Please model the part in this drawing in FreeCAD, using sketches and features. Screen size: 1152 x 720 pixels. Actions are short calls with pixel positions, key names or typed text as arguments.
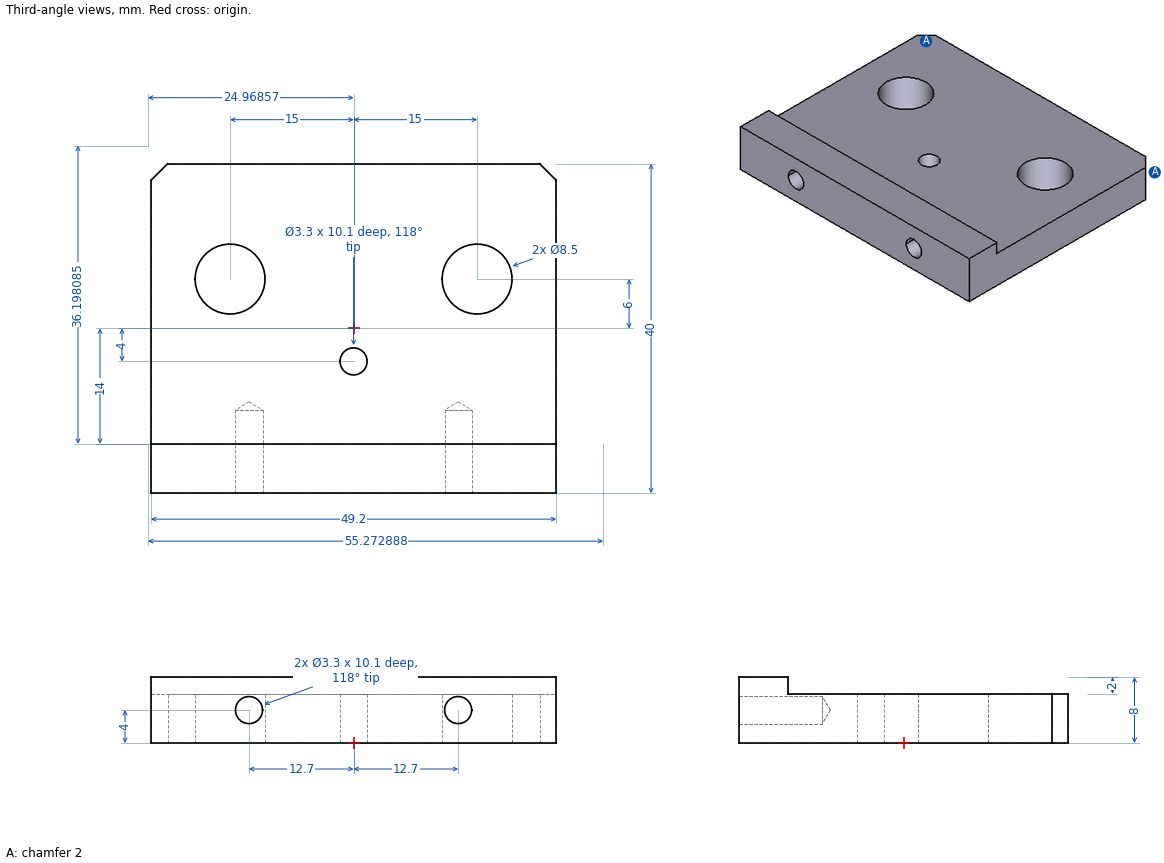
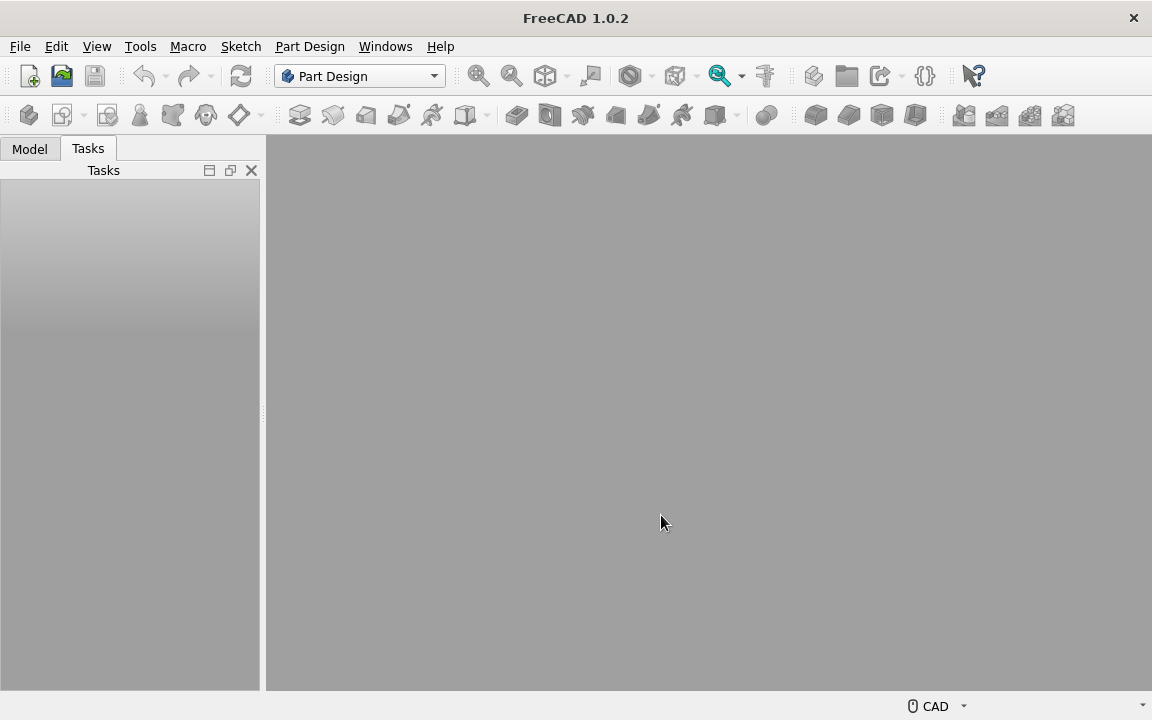
key(ctrl+n)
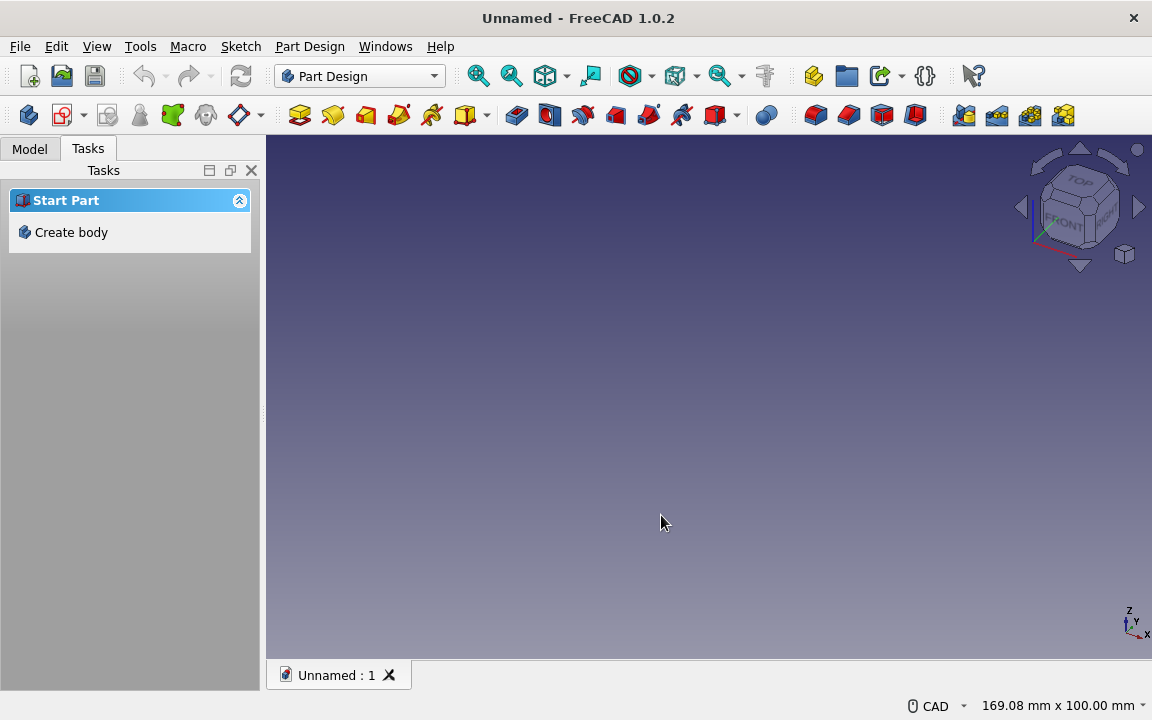
click(62, 116)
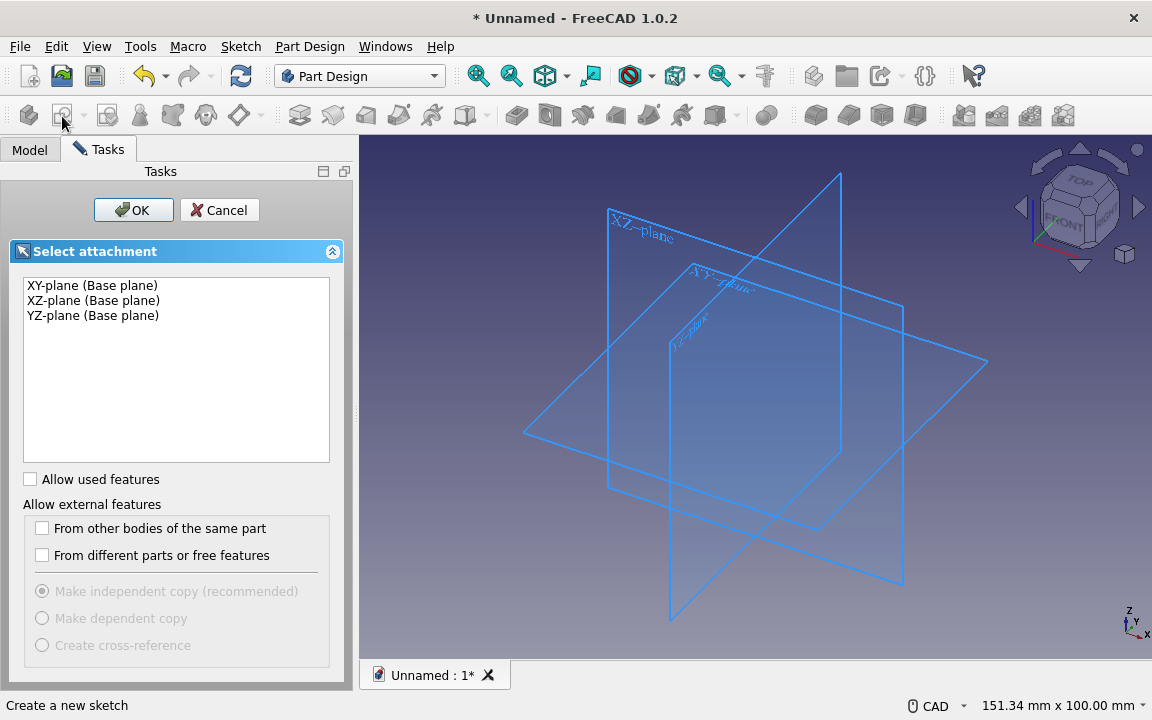
click(84, 286)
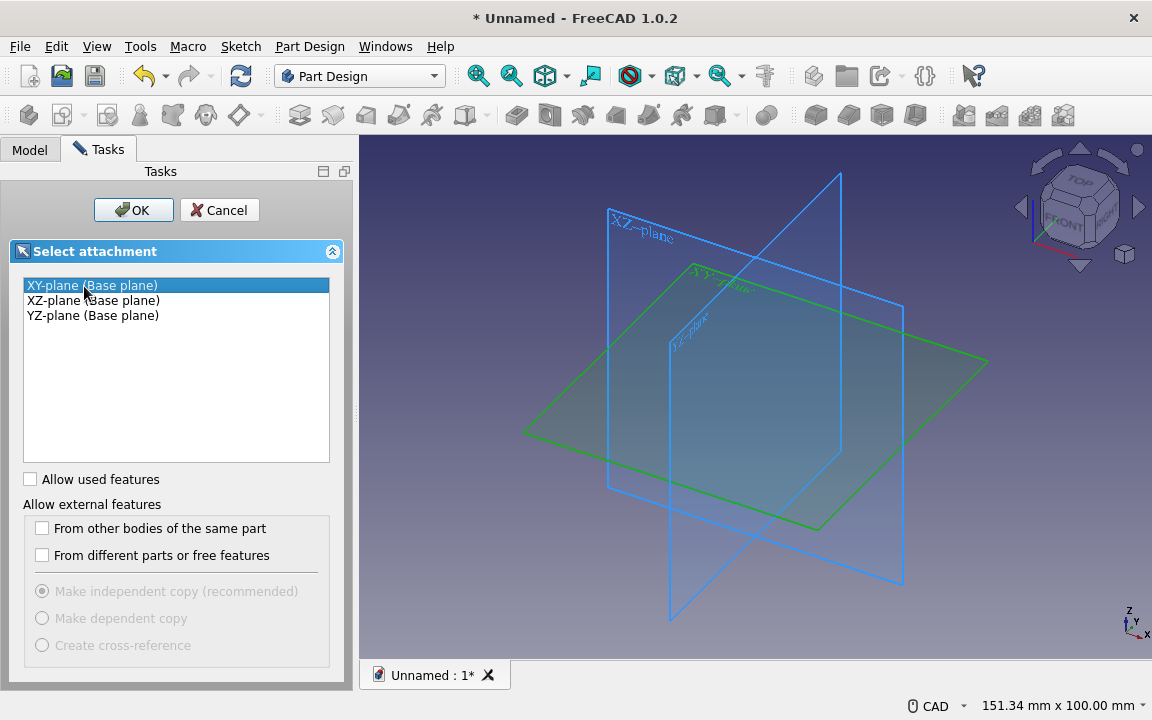
click(134, 210)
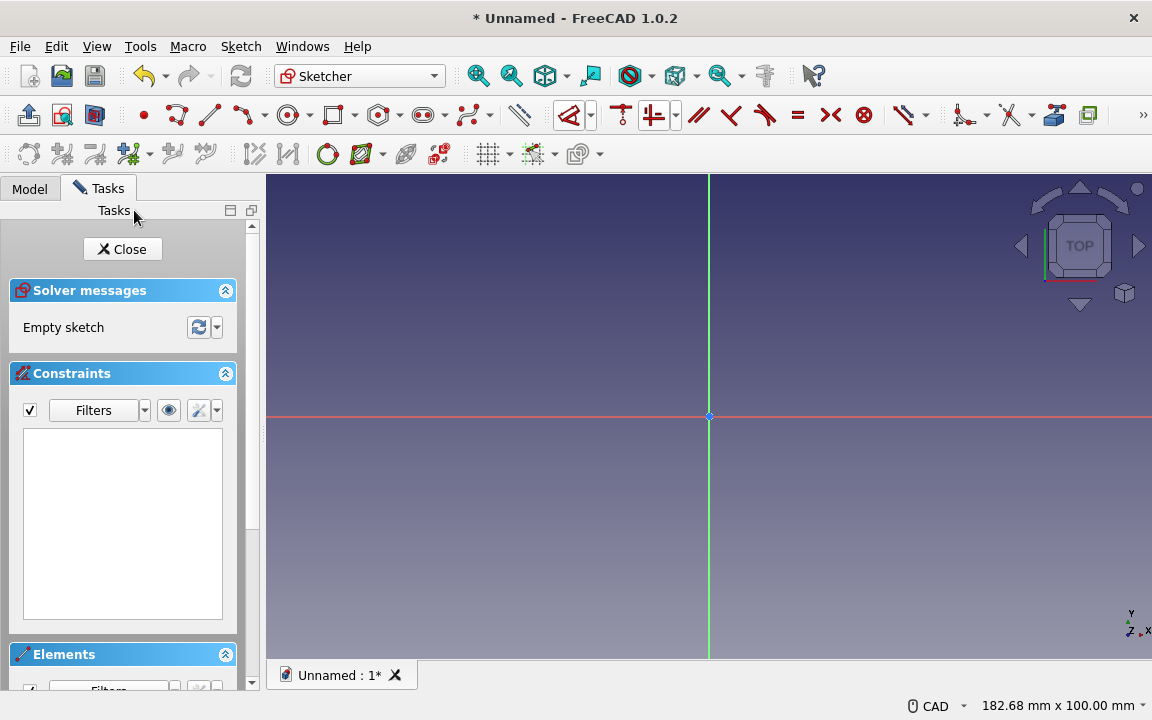
scroll(848, 416, up, 2)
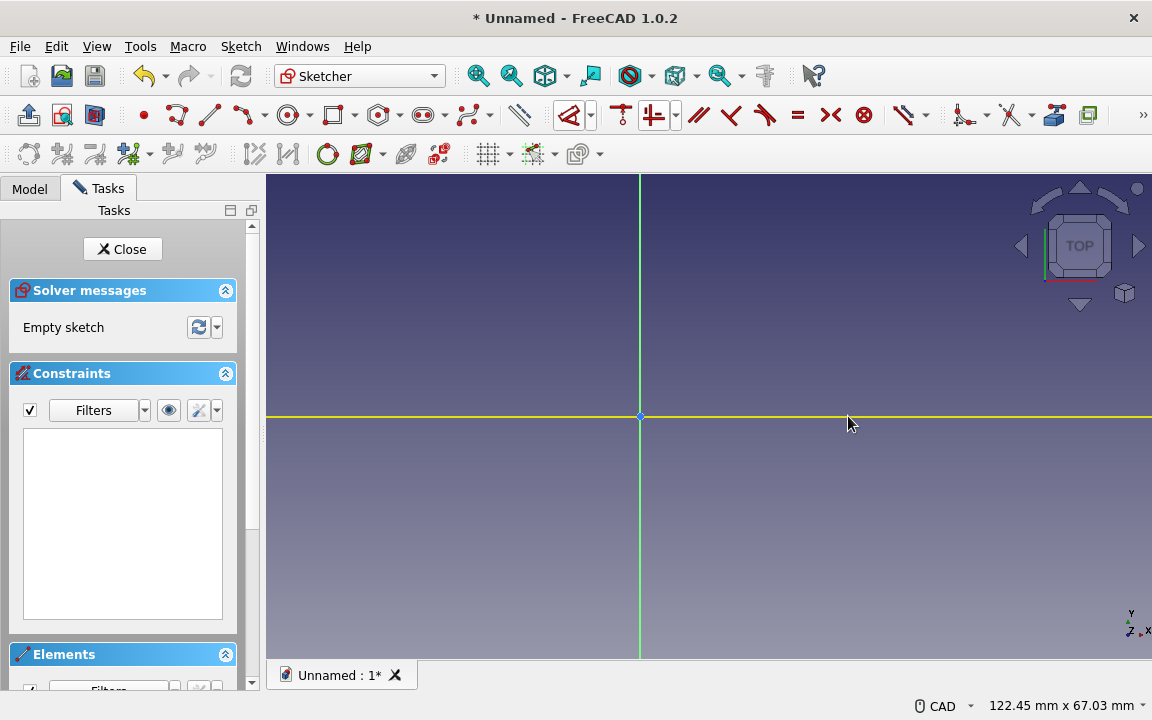
click(354, 116)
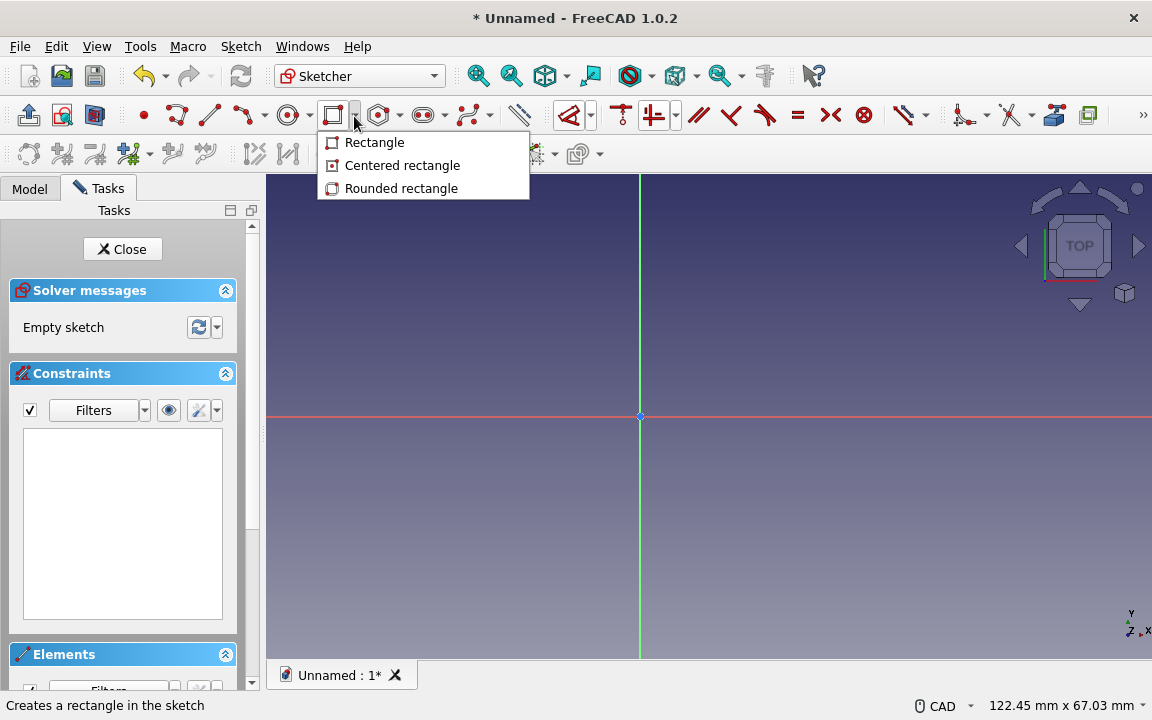
click(424, 166)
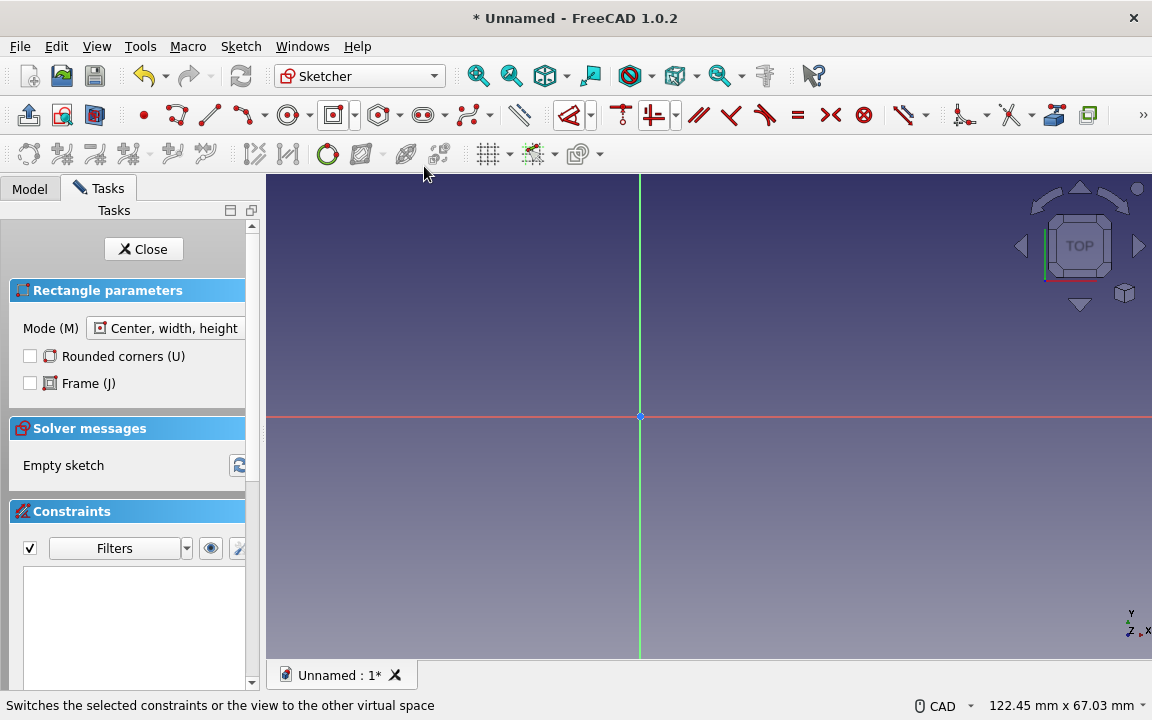
click(640, 416)
click(818, 272)
key(Escape)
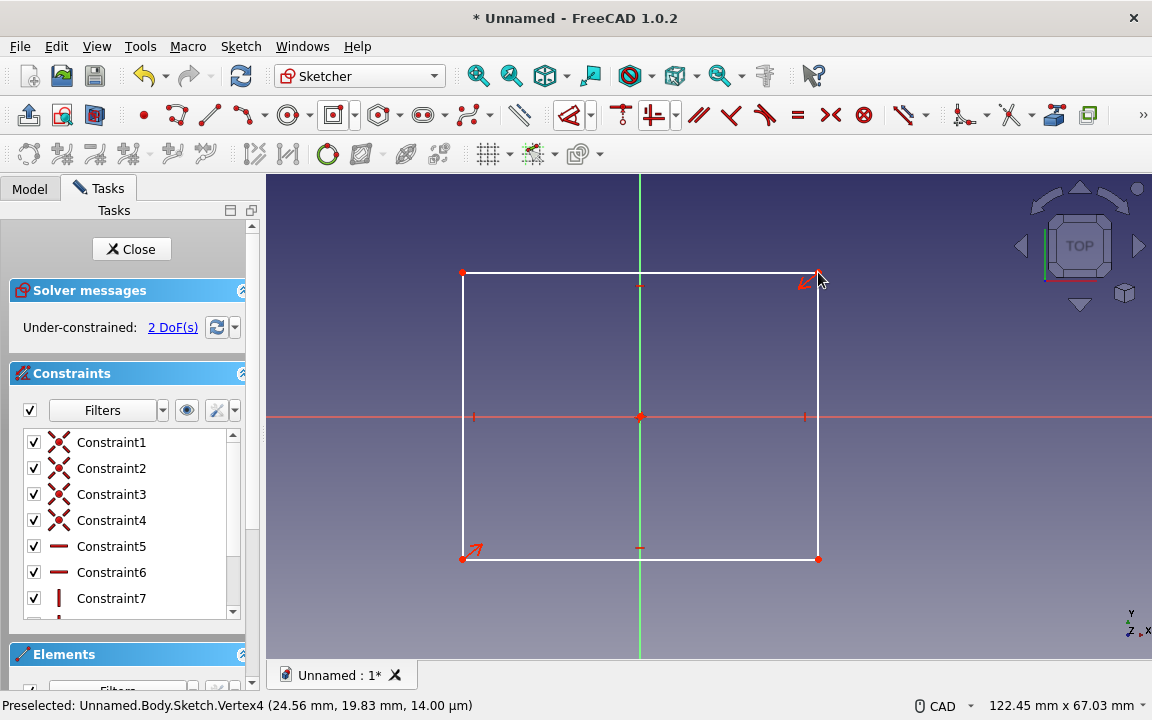
click(568, 116)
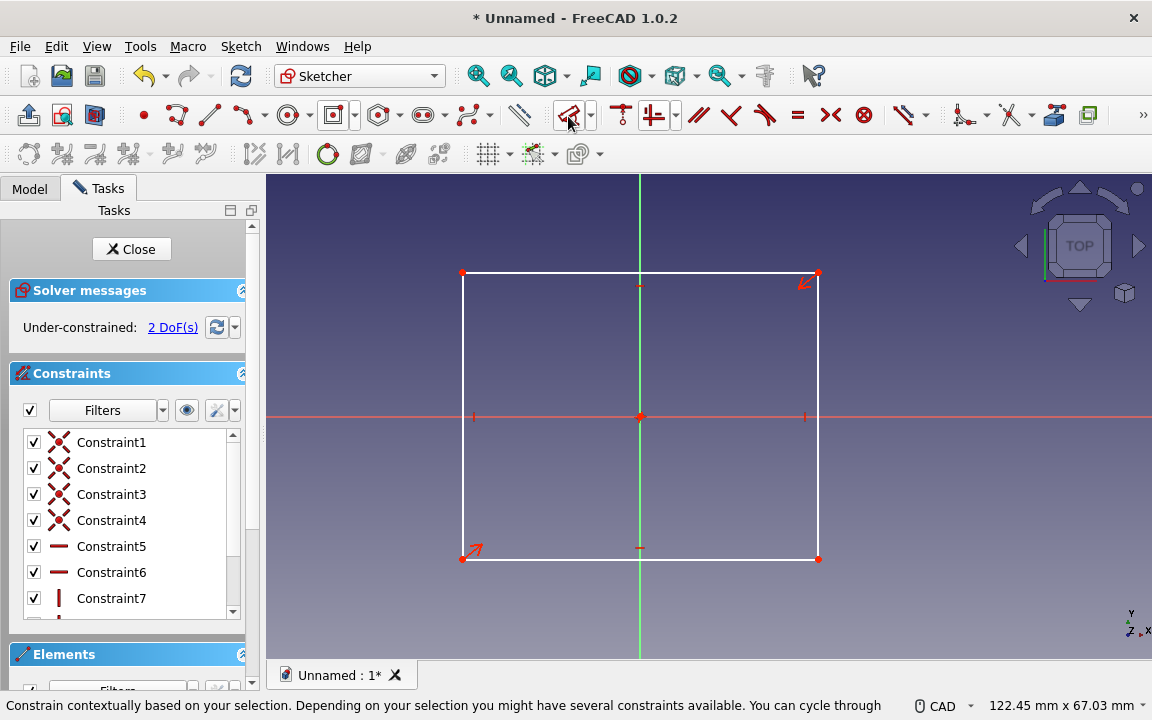
click(818, 474)
click(852, 350)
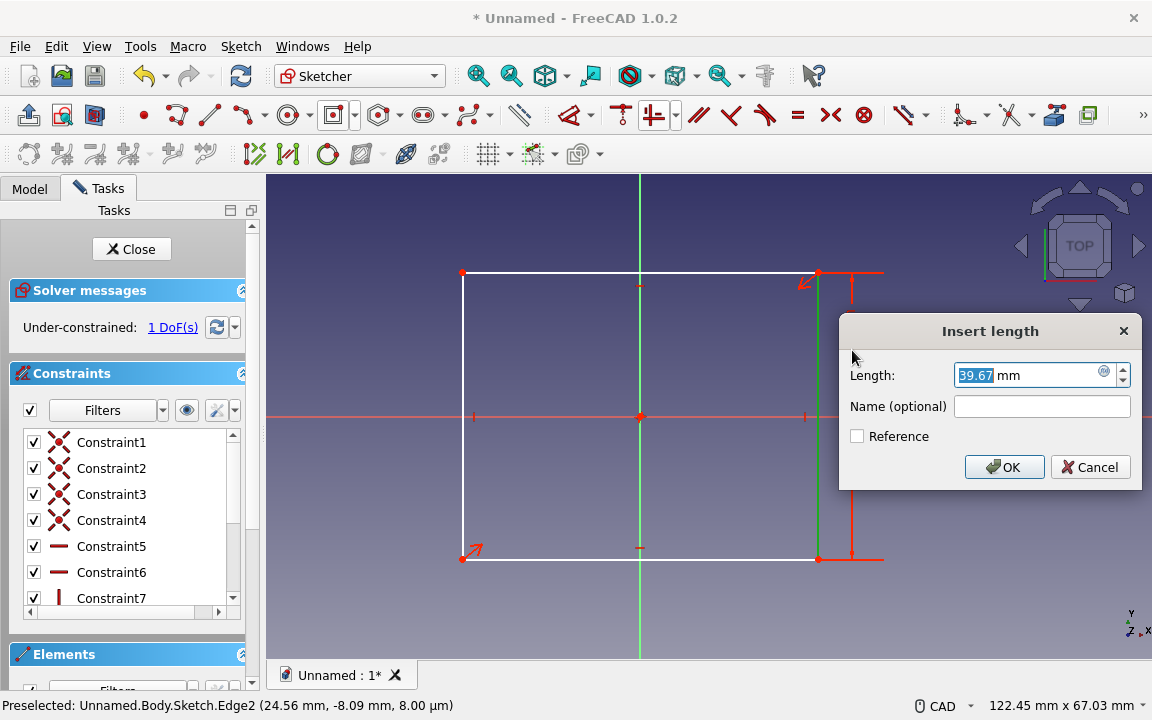
text(40)
key(Return)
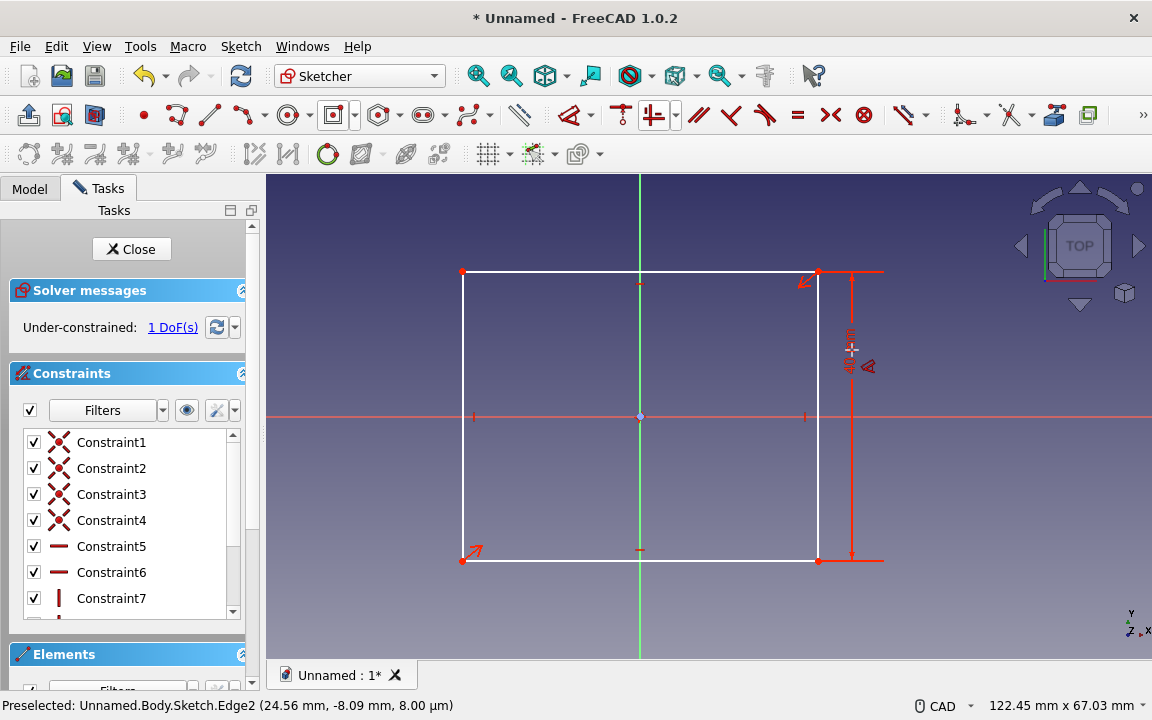
click(569, 561)
click(559, 595)